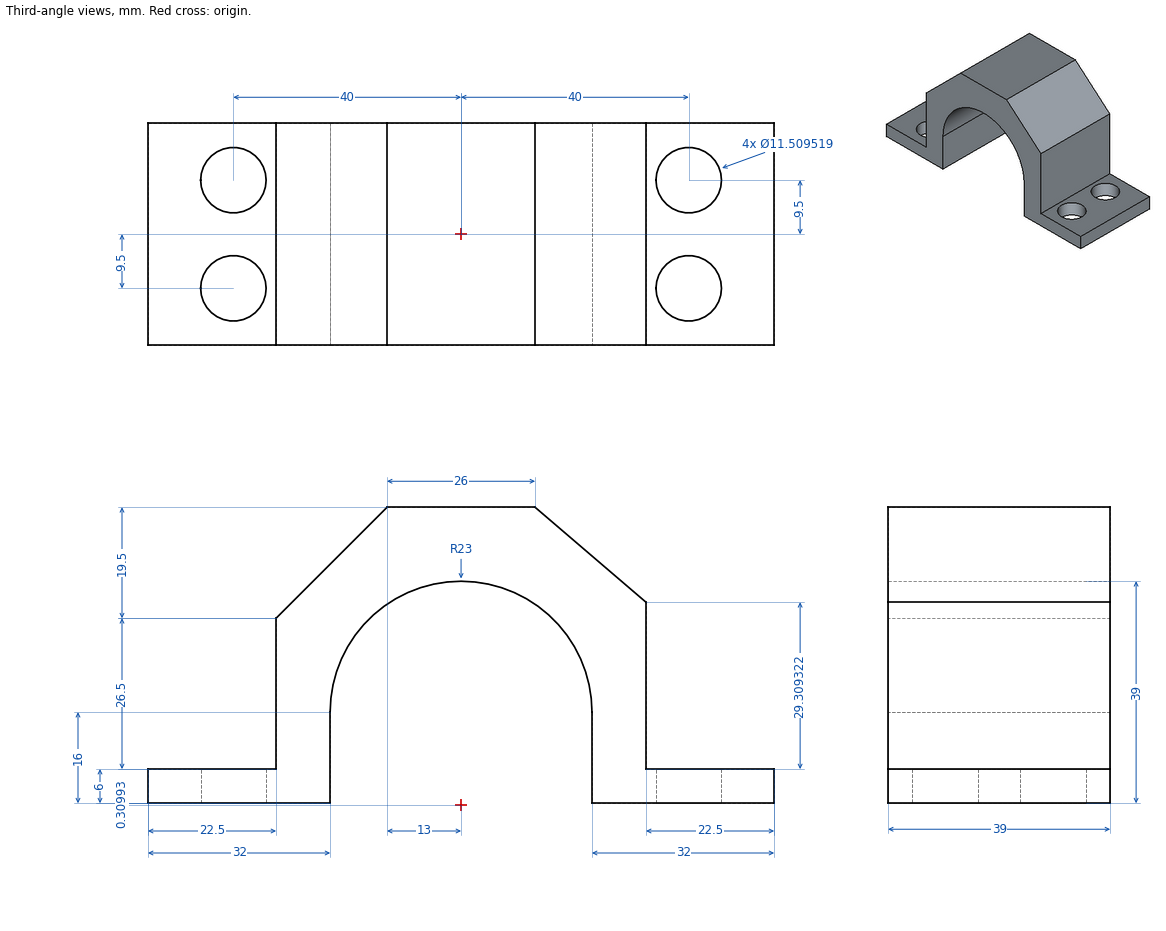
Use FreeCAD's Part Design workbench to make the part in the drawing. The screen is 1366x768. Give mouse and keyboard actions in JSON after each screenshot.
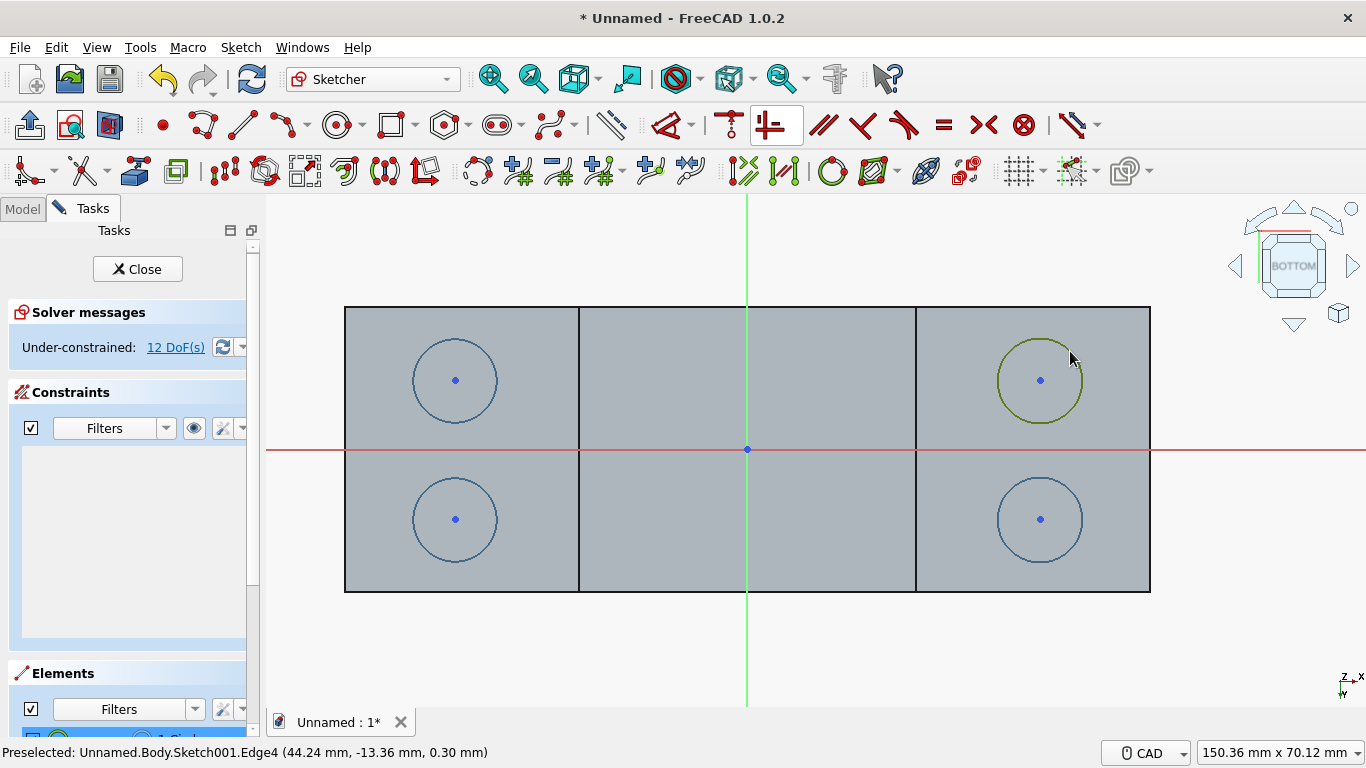
{"action": "left_click", "coordinate": [944, 126]}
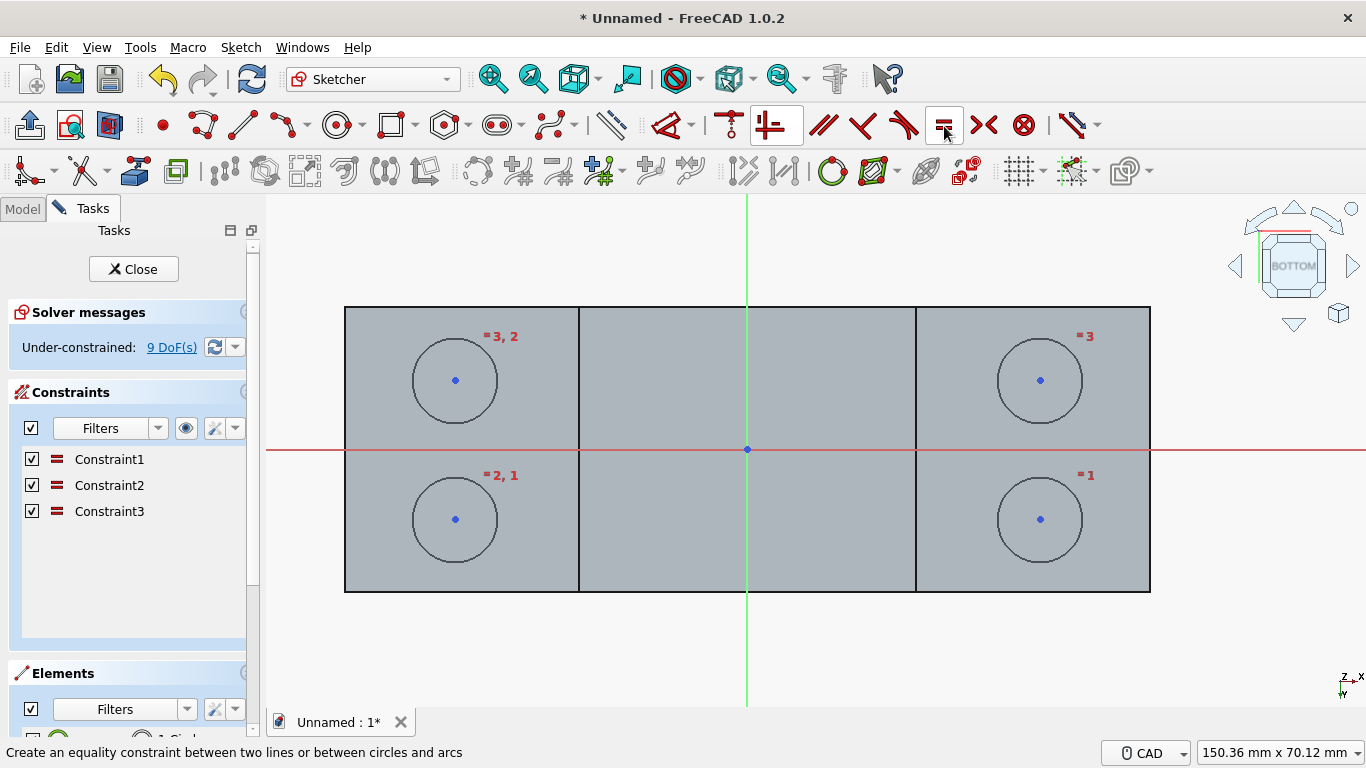
{"action": "left_click", "coordinate": [1040, 520]}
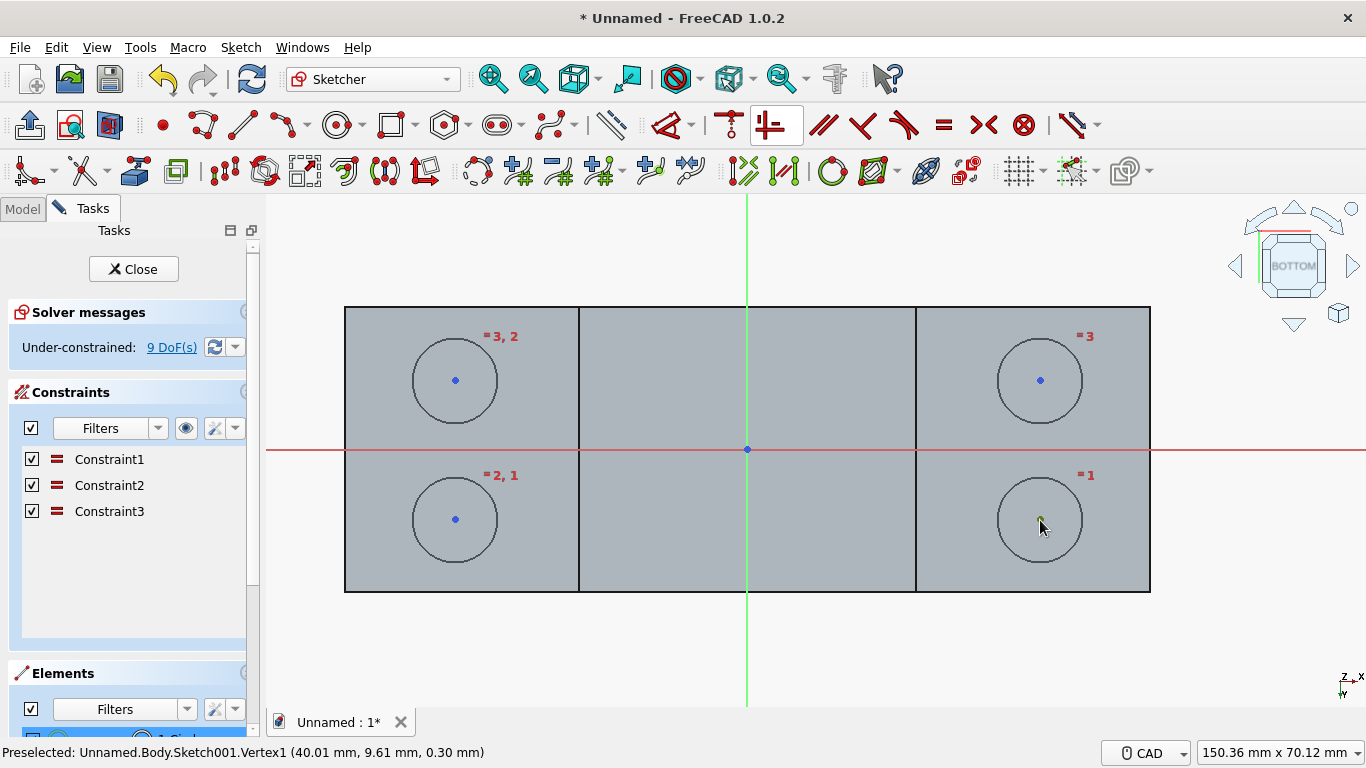
{"action": "left_click", "coordinate": [455, 520]}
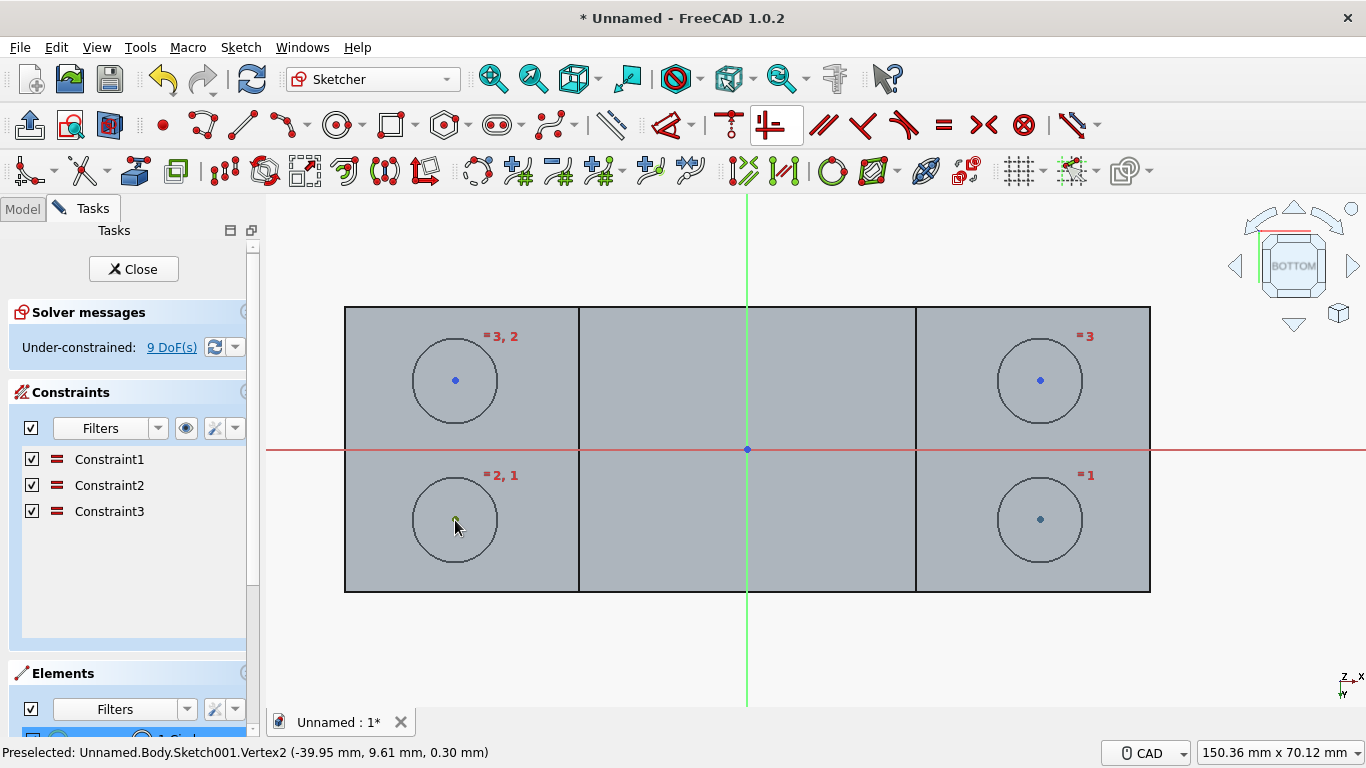
{"action": "key", "text": "h"}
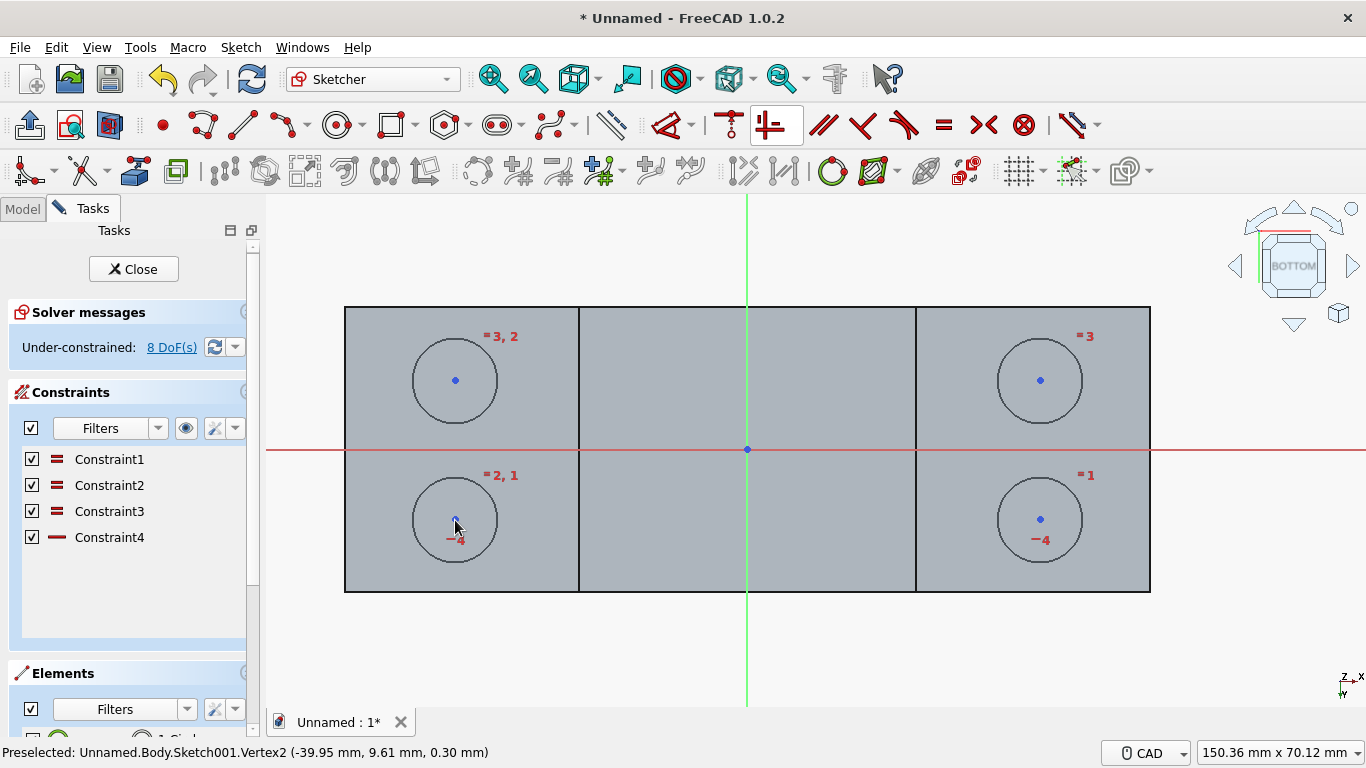
{"action": "left_click", "coordinate": [455, 520]}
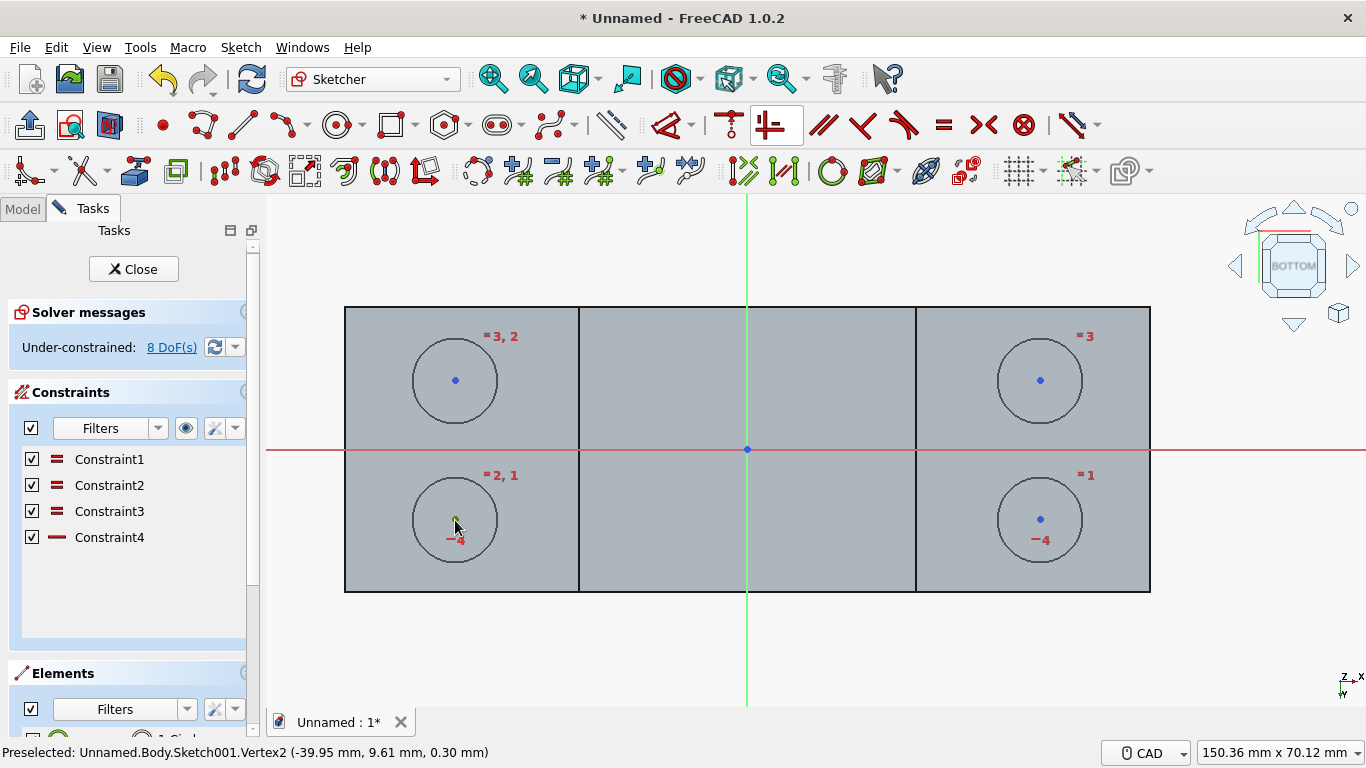
{"action": "left_click", "coordinate": [455, 381]}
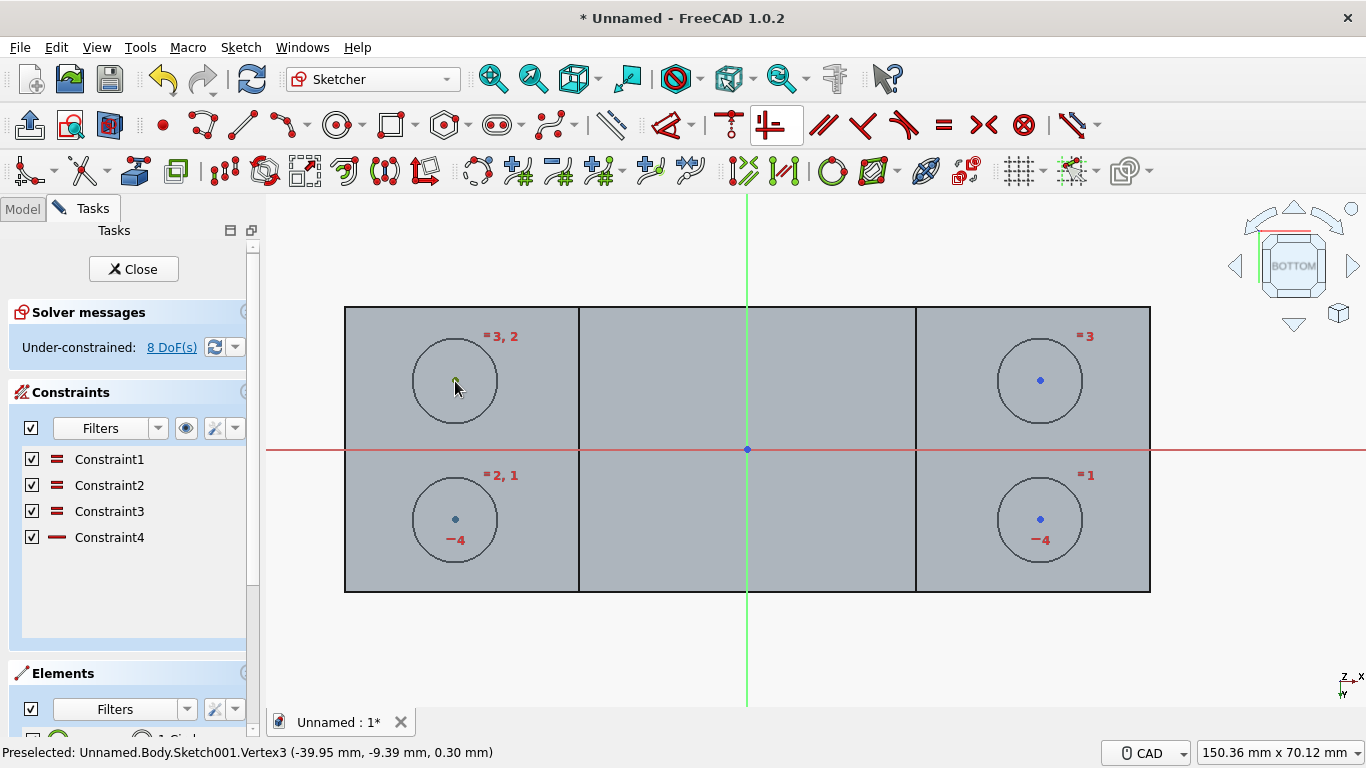
{"action": "key", "text": "v"}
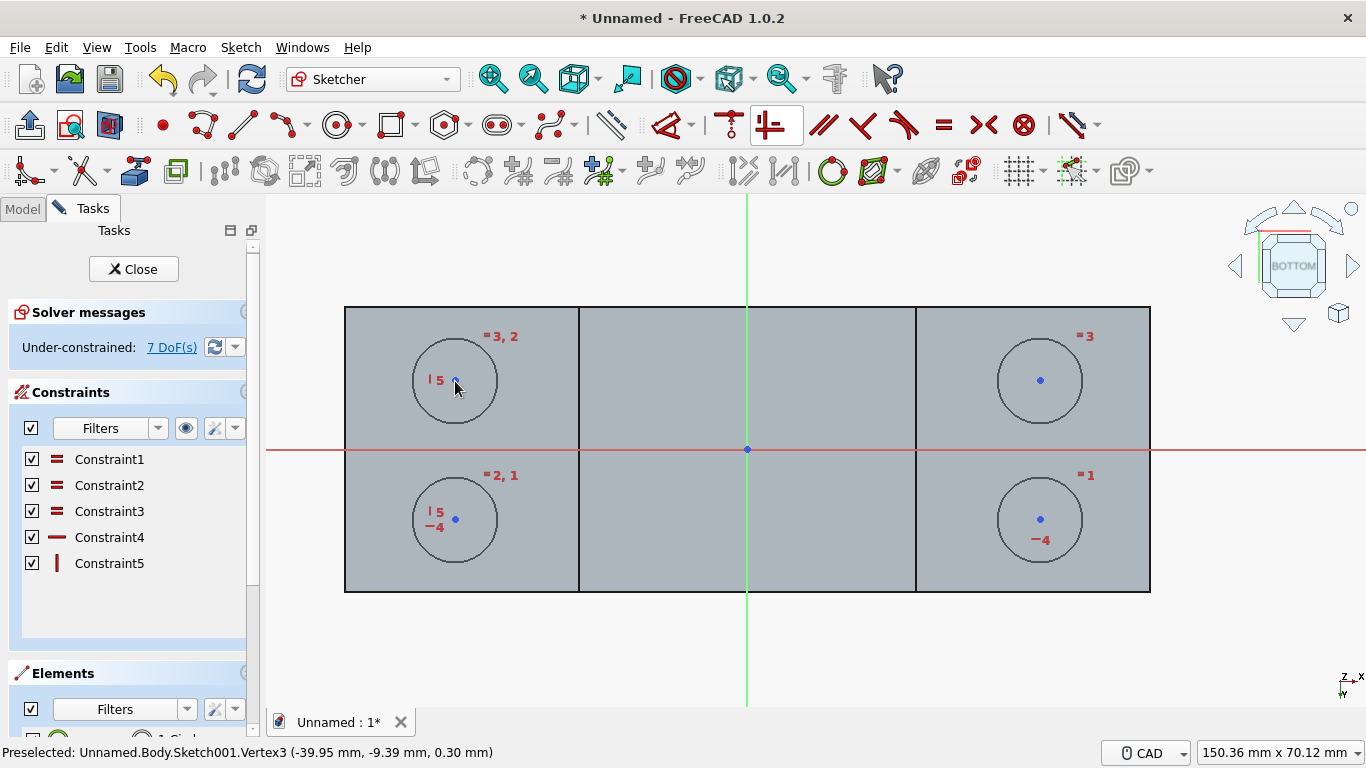
{"action": "left_click", "coordinate": [1040, 520]}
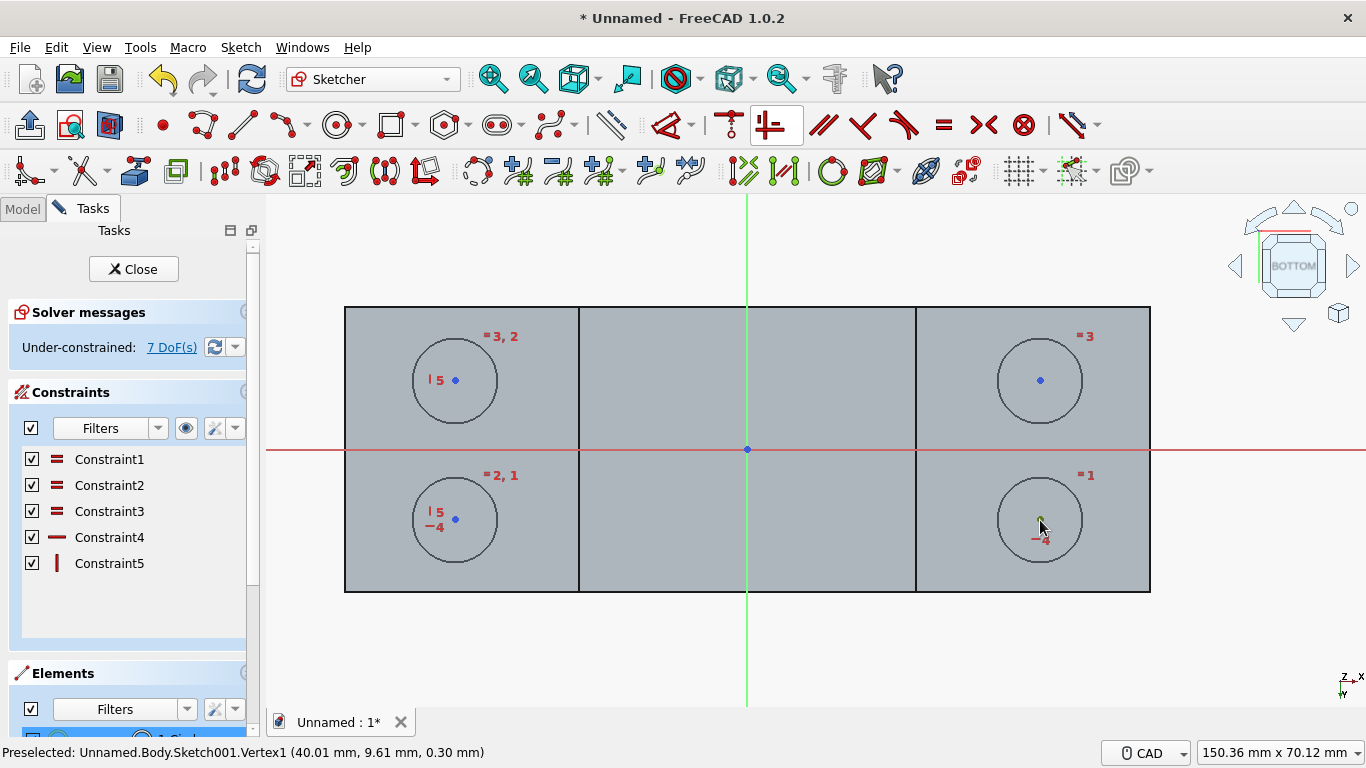
{"action": "left_click", "coordinate": [1040, 381]}